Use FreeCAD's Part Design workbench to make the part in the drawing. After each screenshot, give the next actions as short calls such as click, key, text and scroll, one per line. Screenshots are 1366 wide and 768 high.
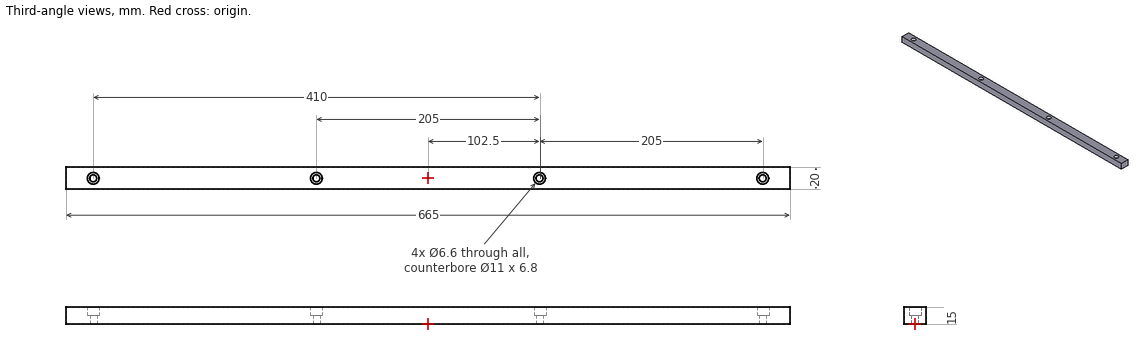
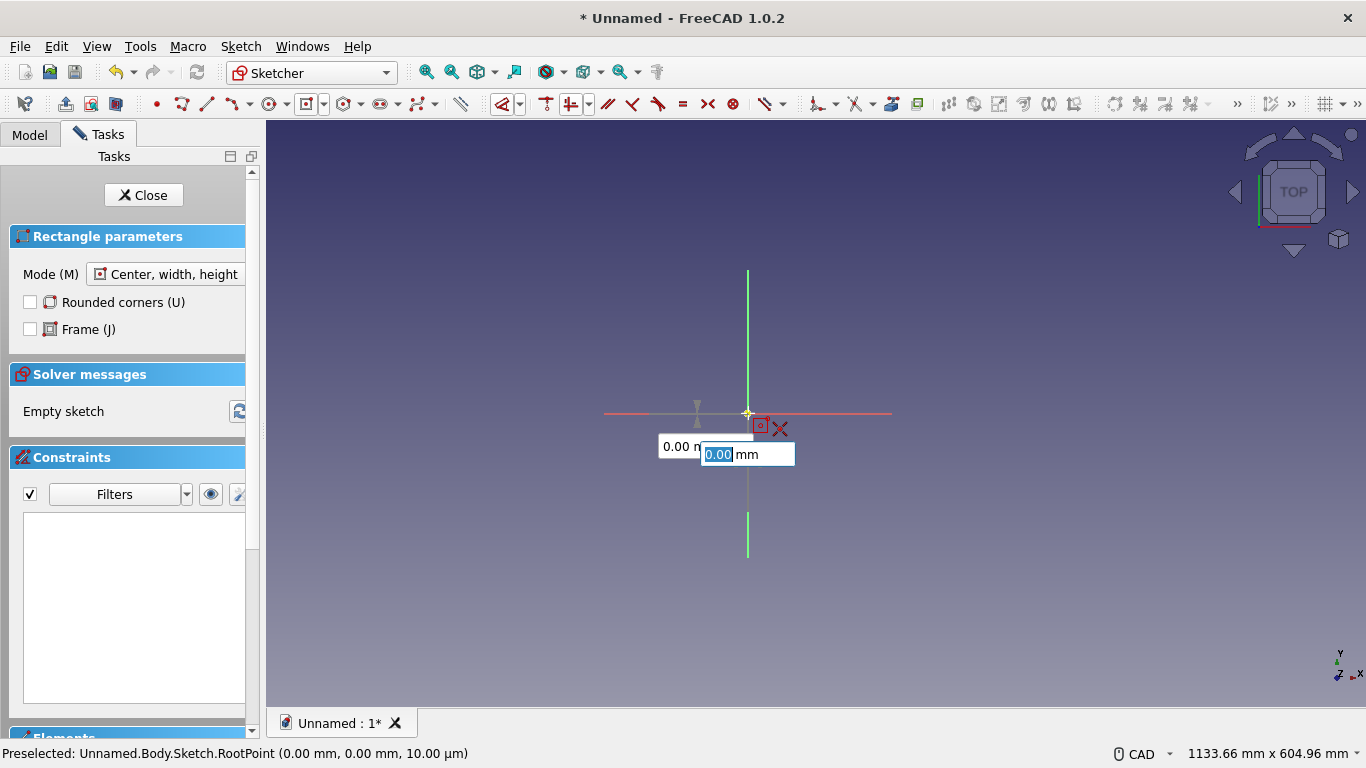
scroll(1071, 404, up, 3)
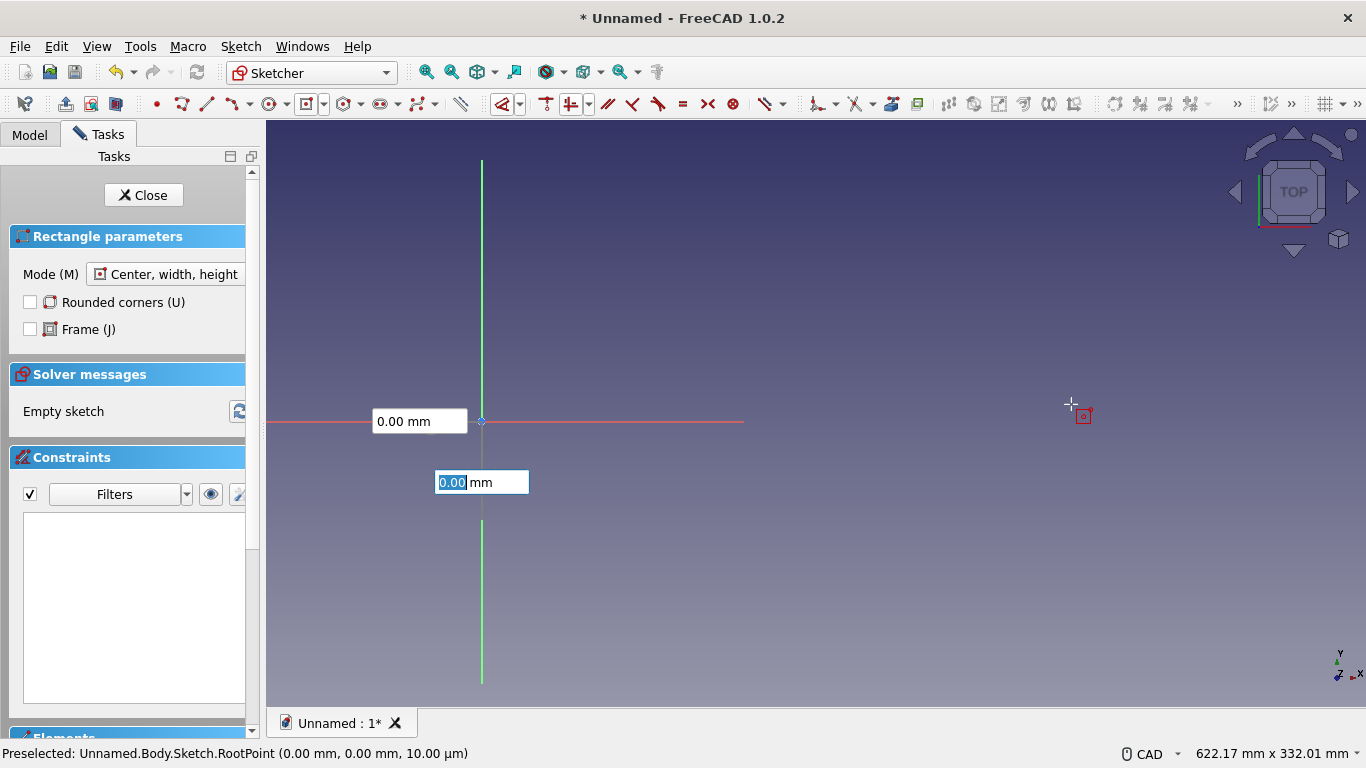
click(1070, 404)
key(Escape)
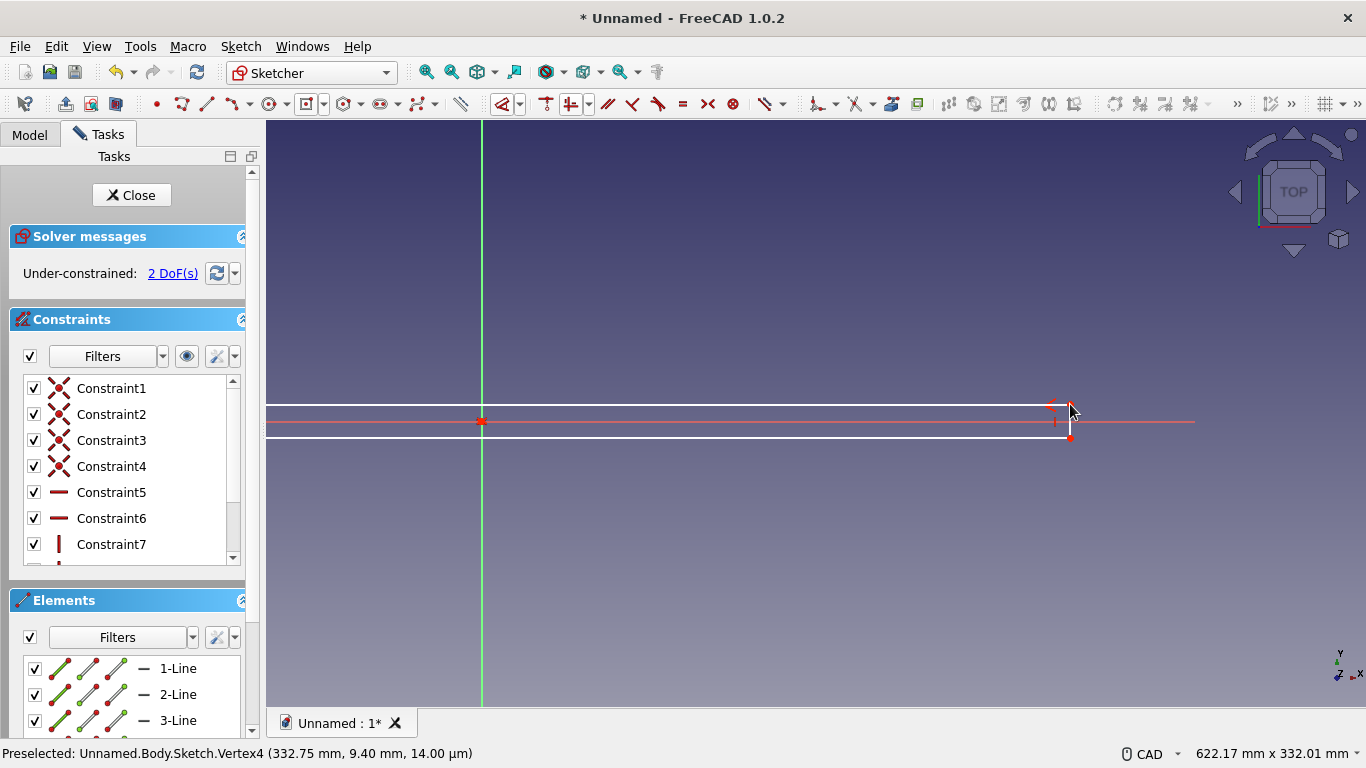
click(1070, 425)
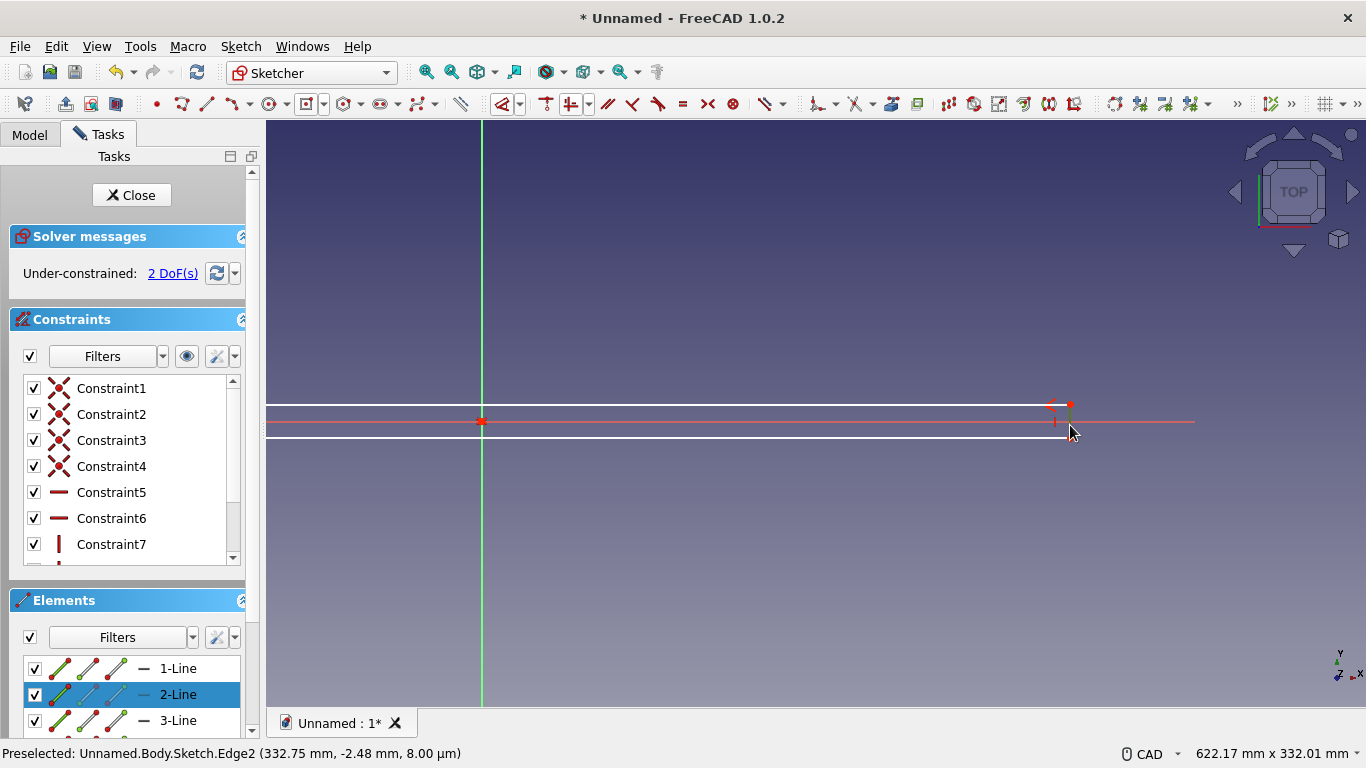
click(520, 104)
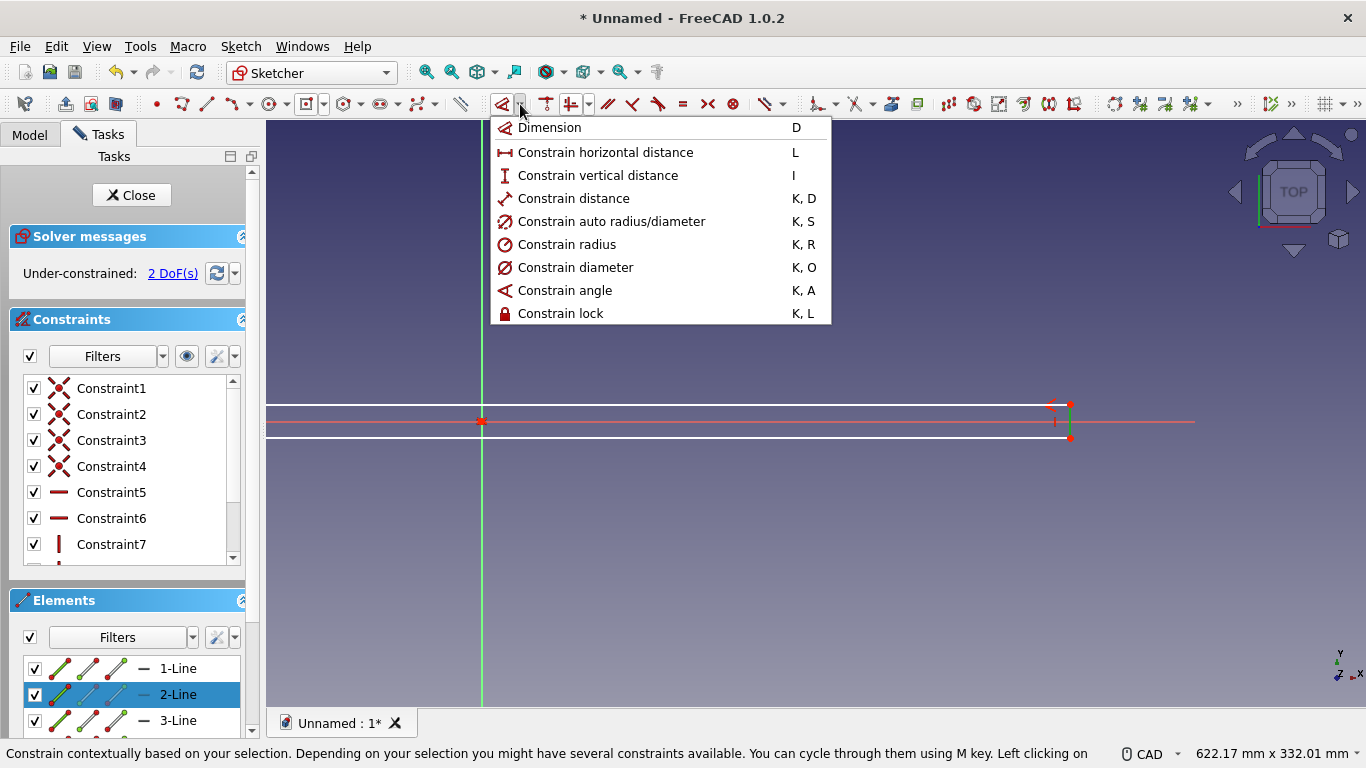
click(661, 176)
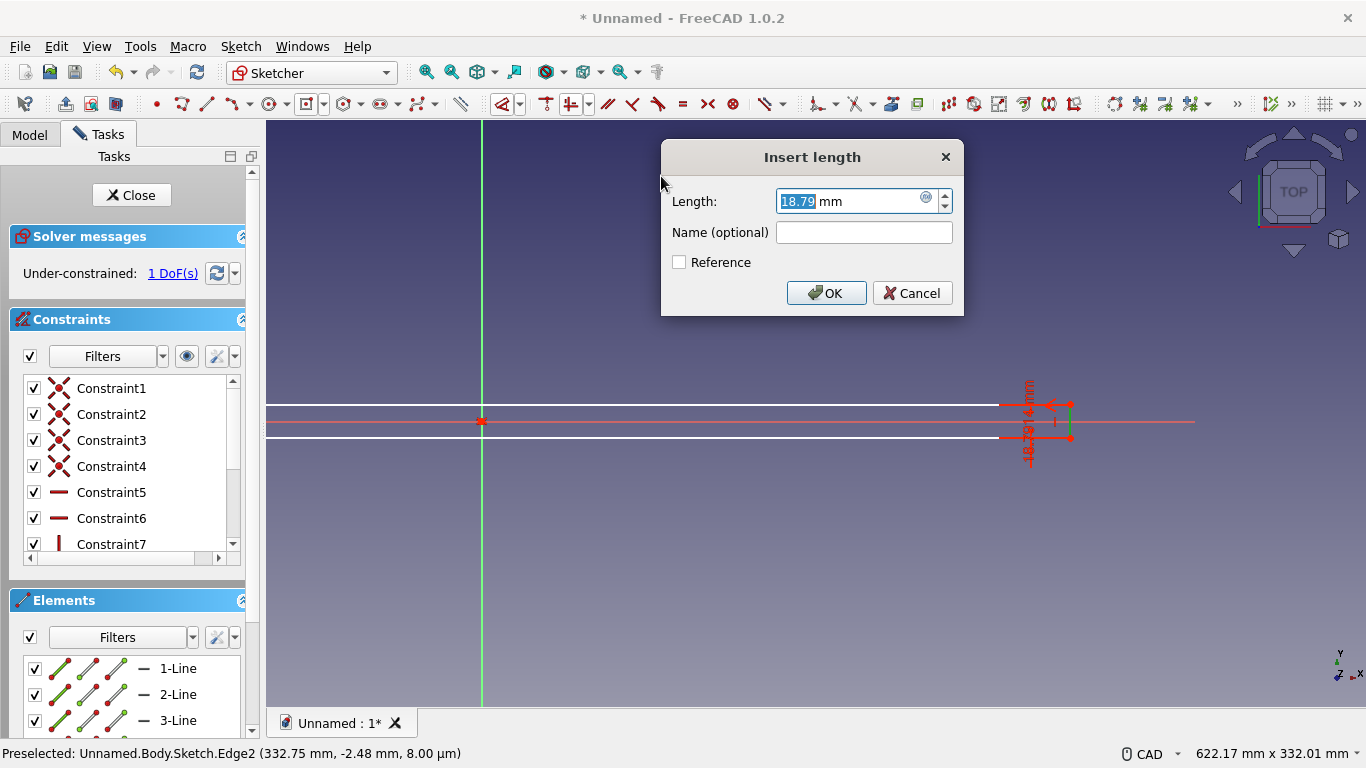
text(20)
key(Return)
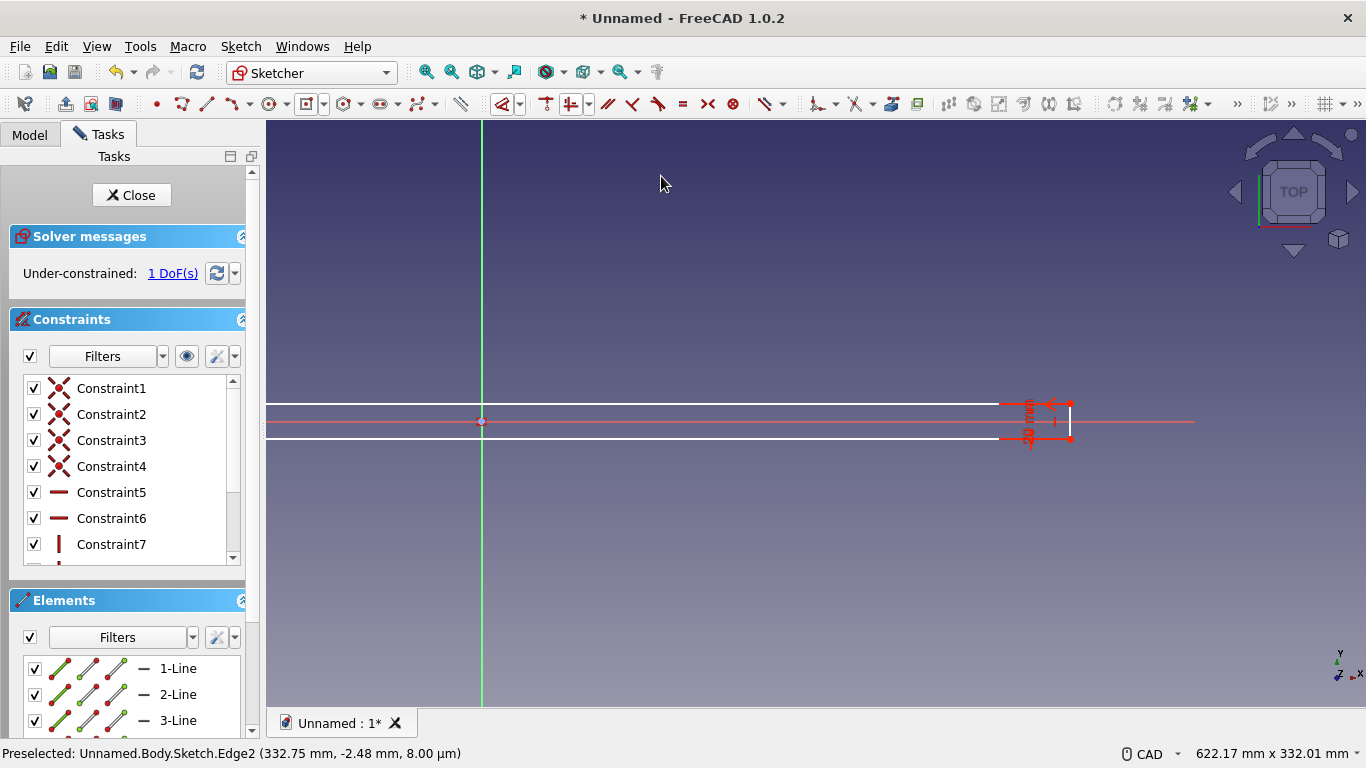
click(717, 439)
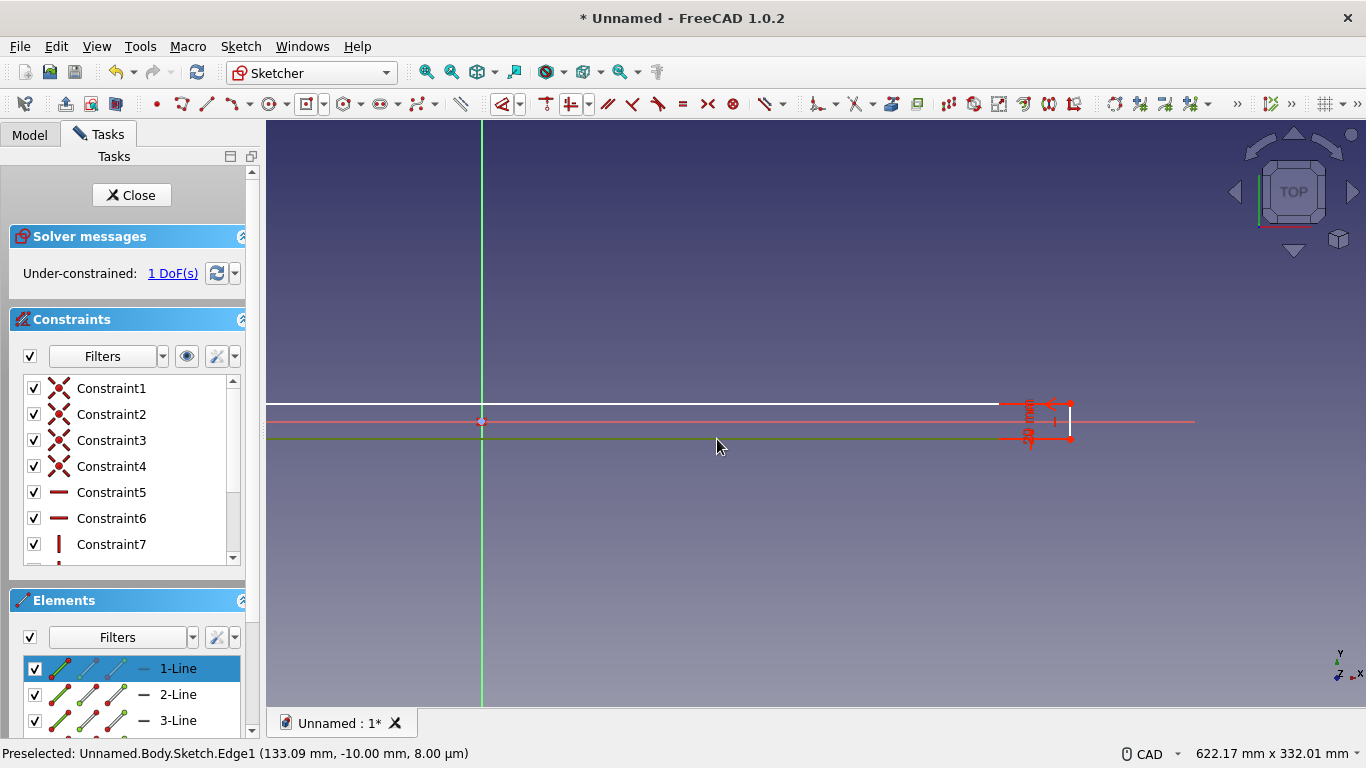
key(l)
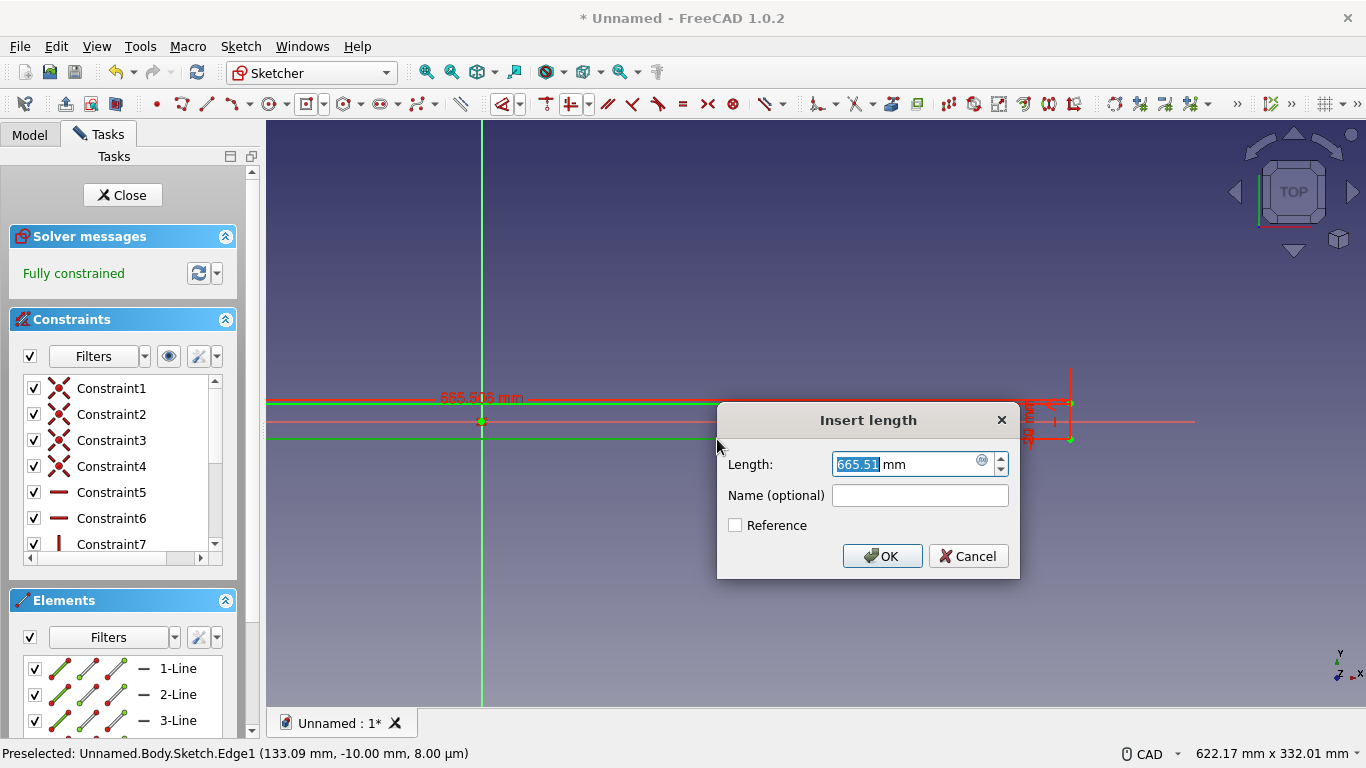
text(665)
key(Return)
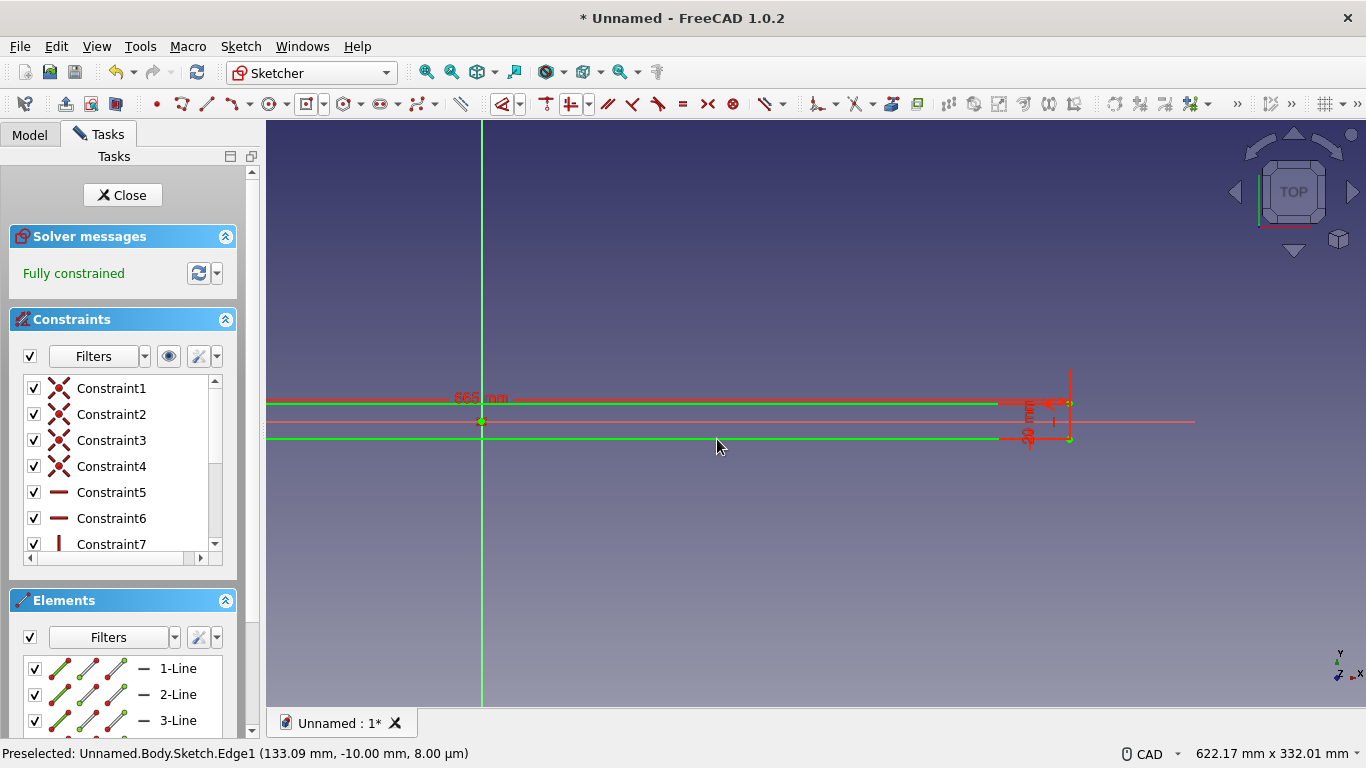
click(123, 195)